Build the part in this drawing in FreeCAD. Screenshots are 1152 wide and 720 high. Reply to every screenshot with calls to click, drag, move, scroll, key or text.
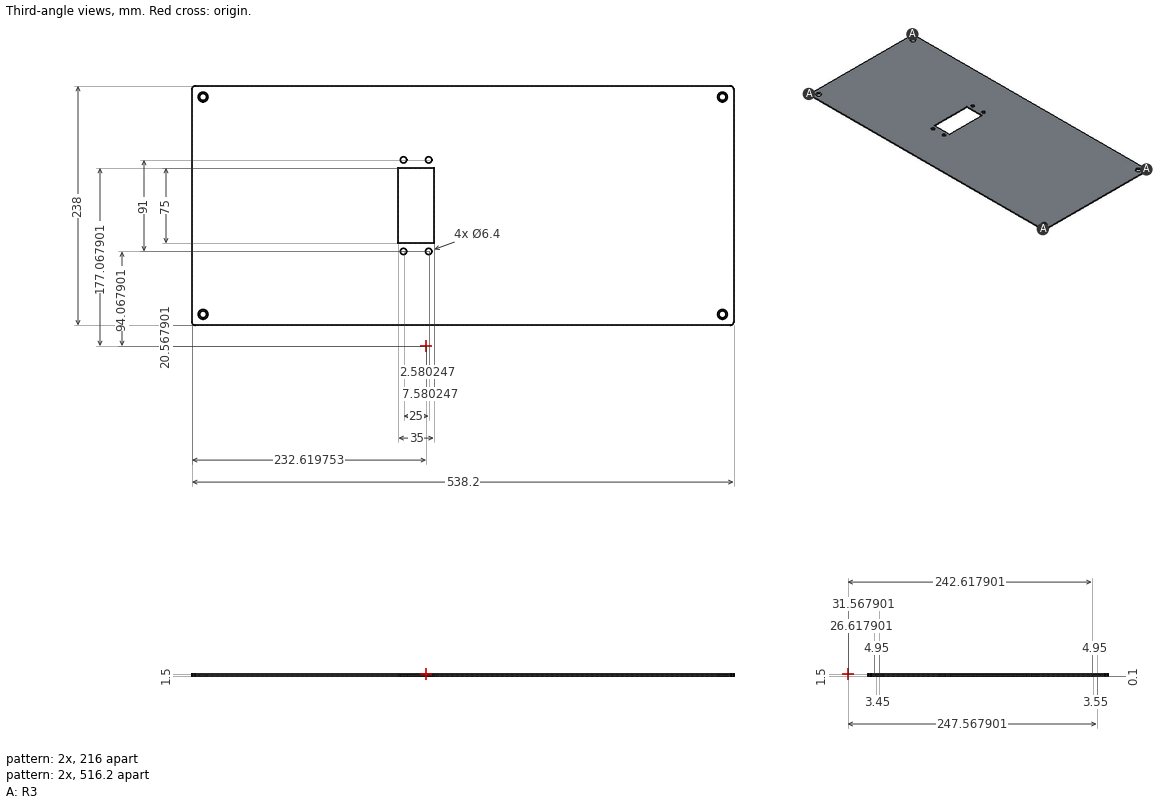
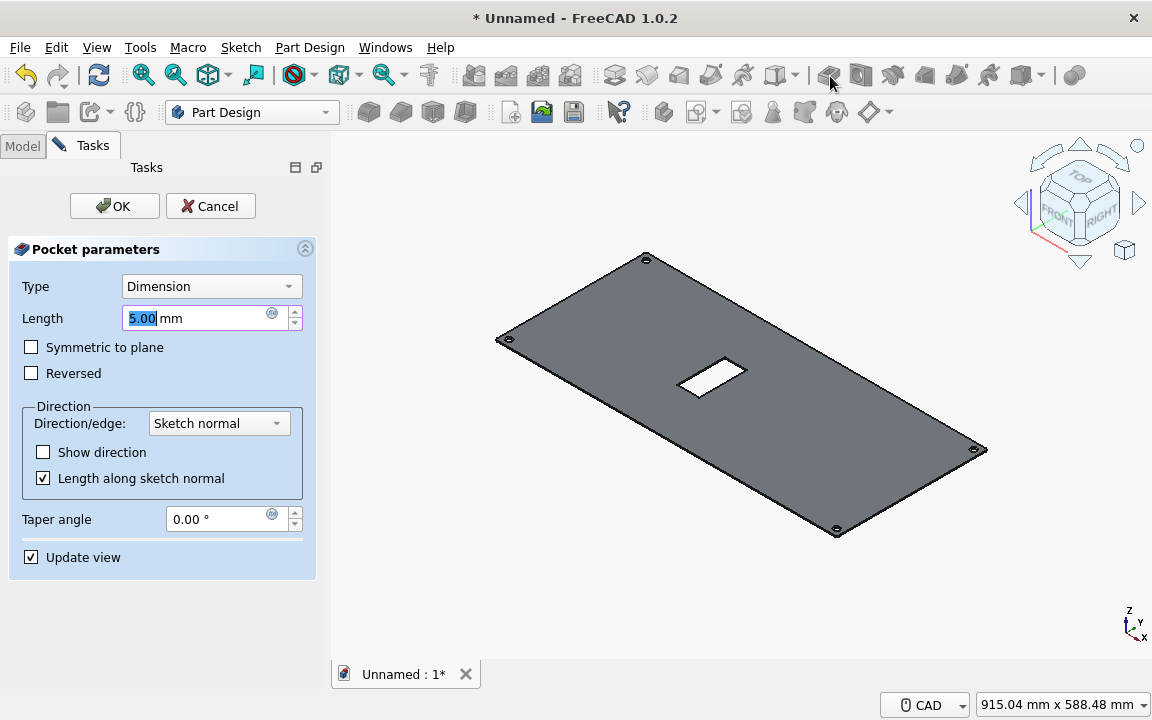
text(1.5)
key(Tab)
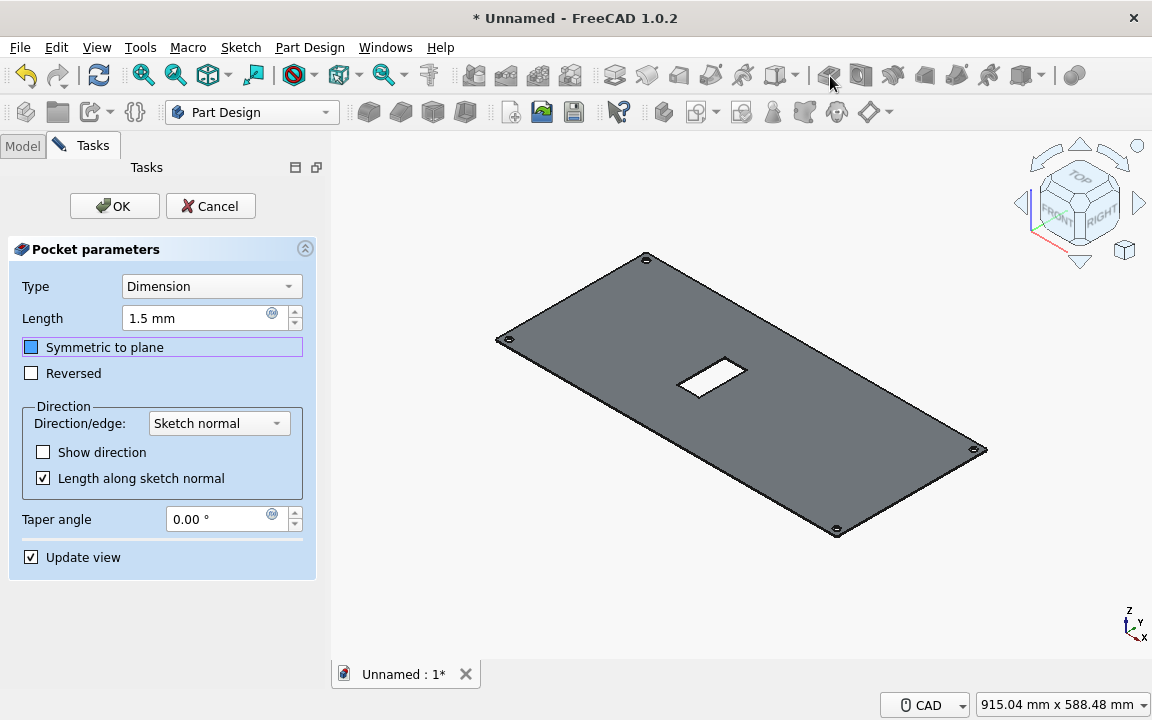
click(115, 206)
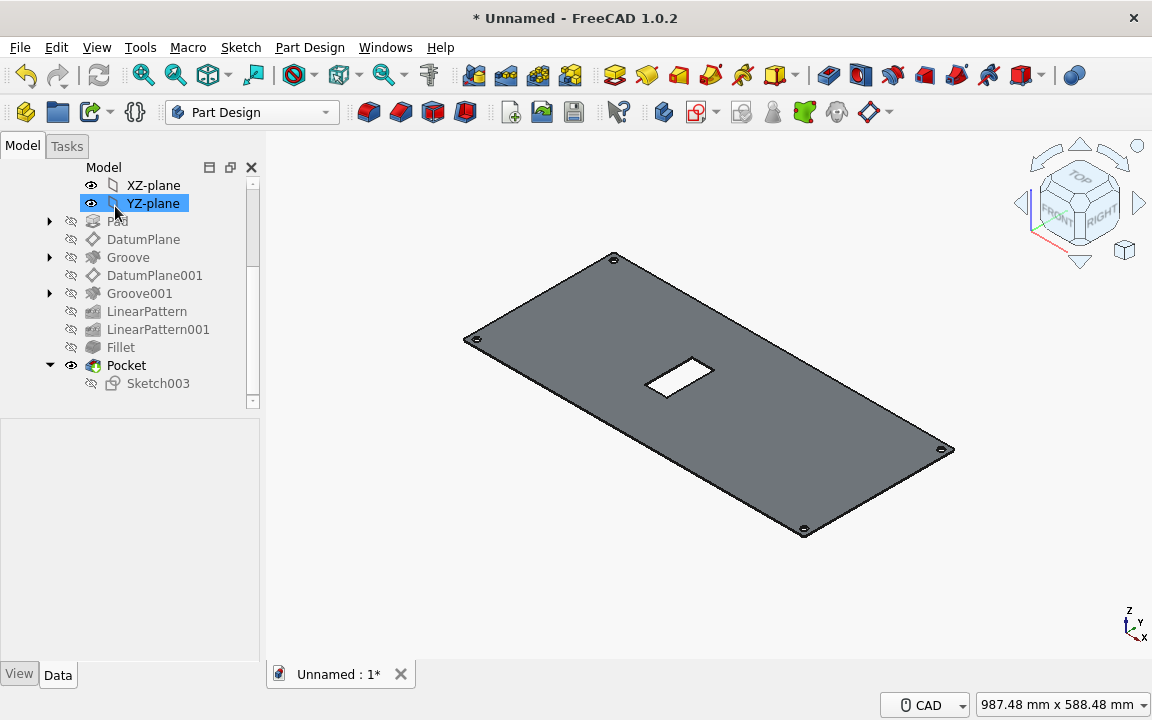
click(807, 450)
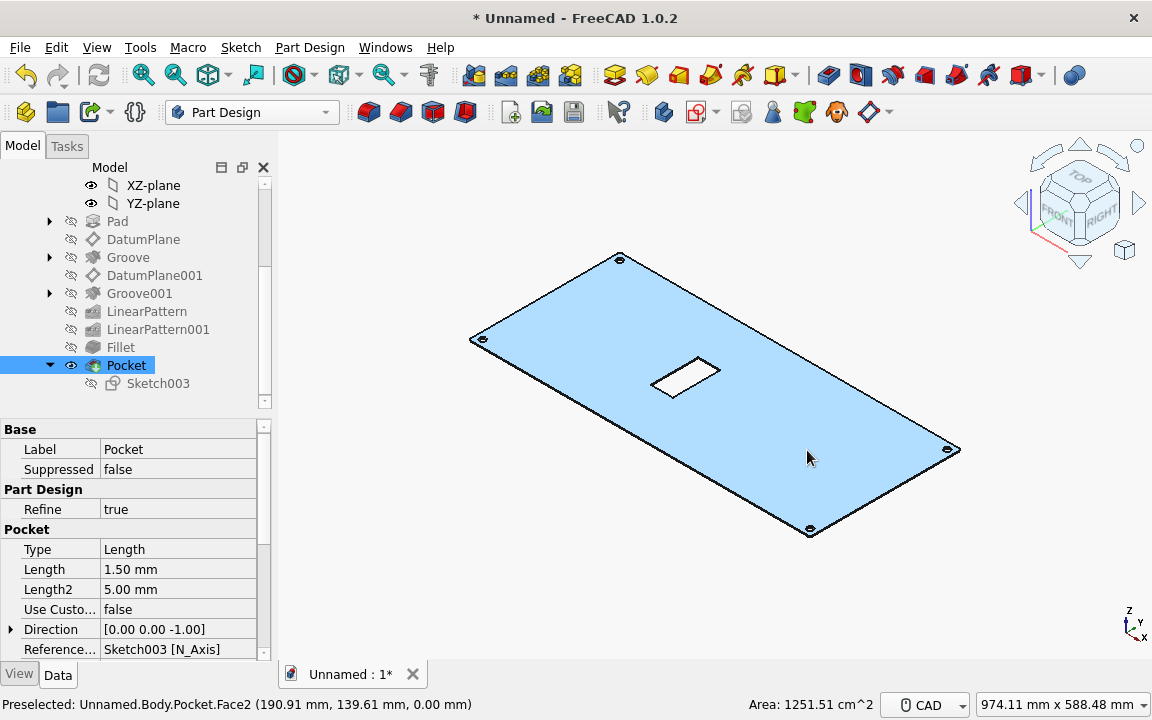
click(696, 112)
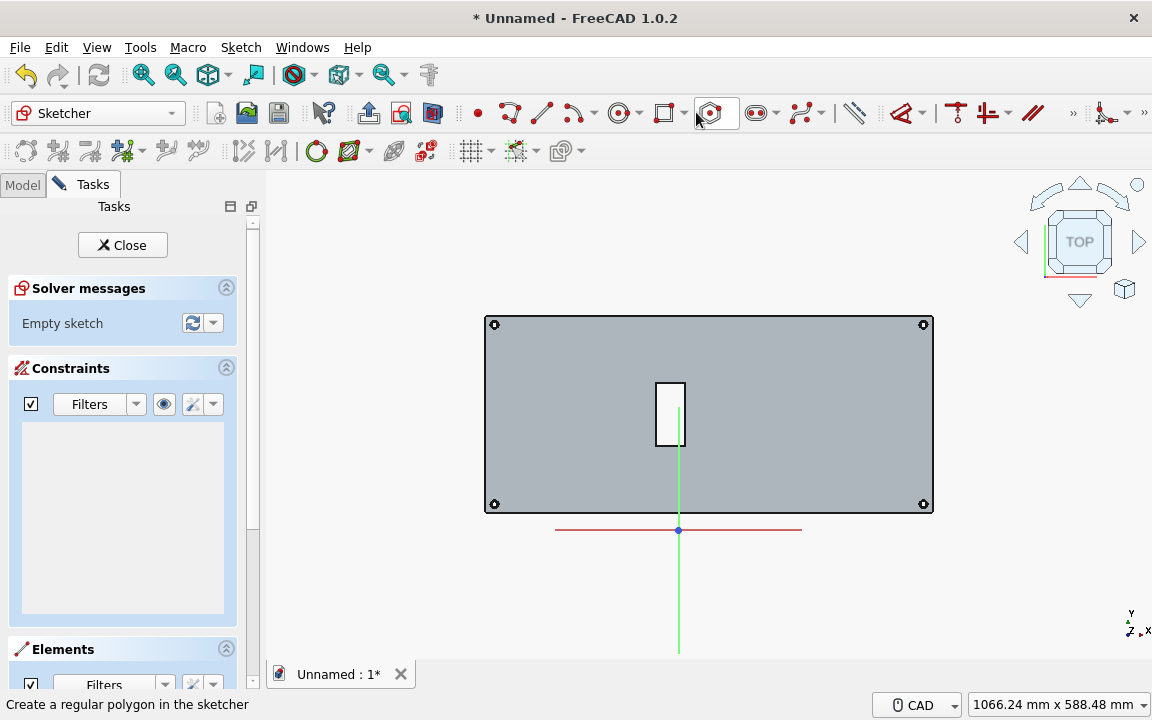
scroll(707, 498, up, 3)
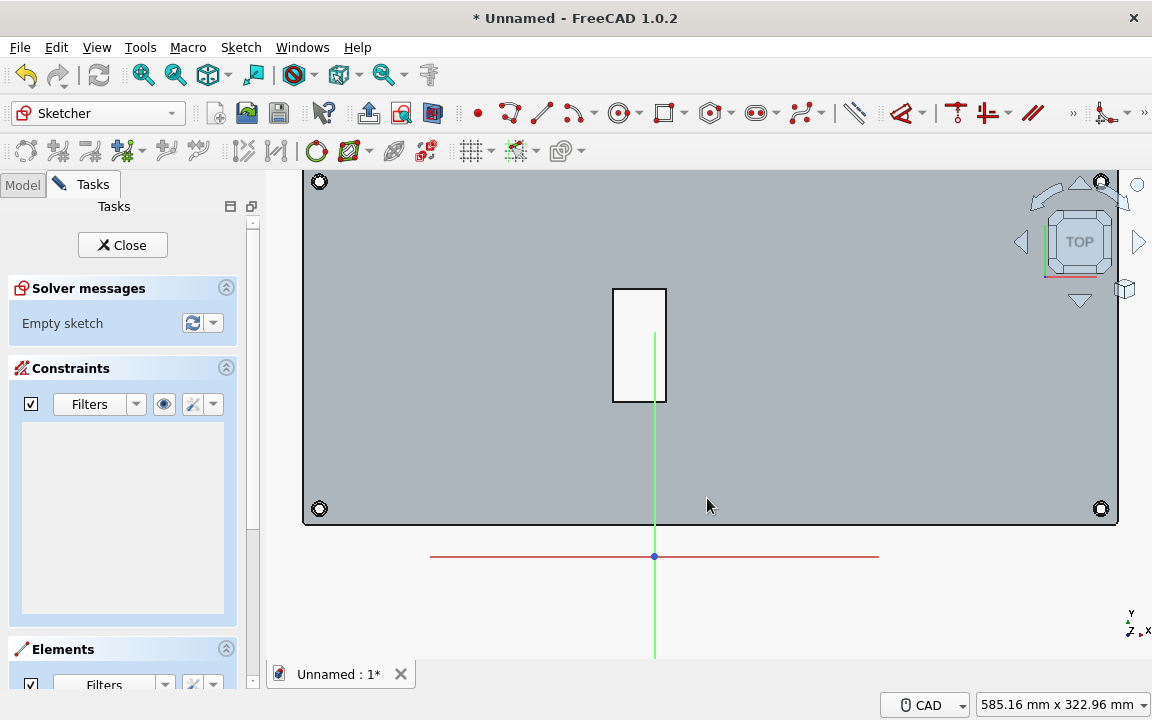
key(g)
key(c)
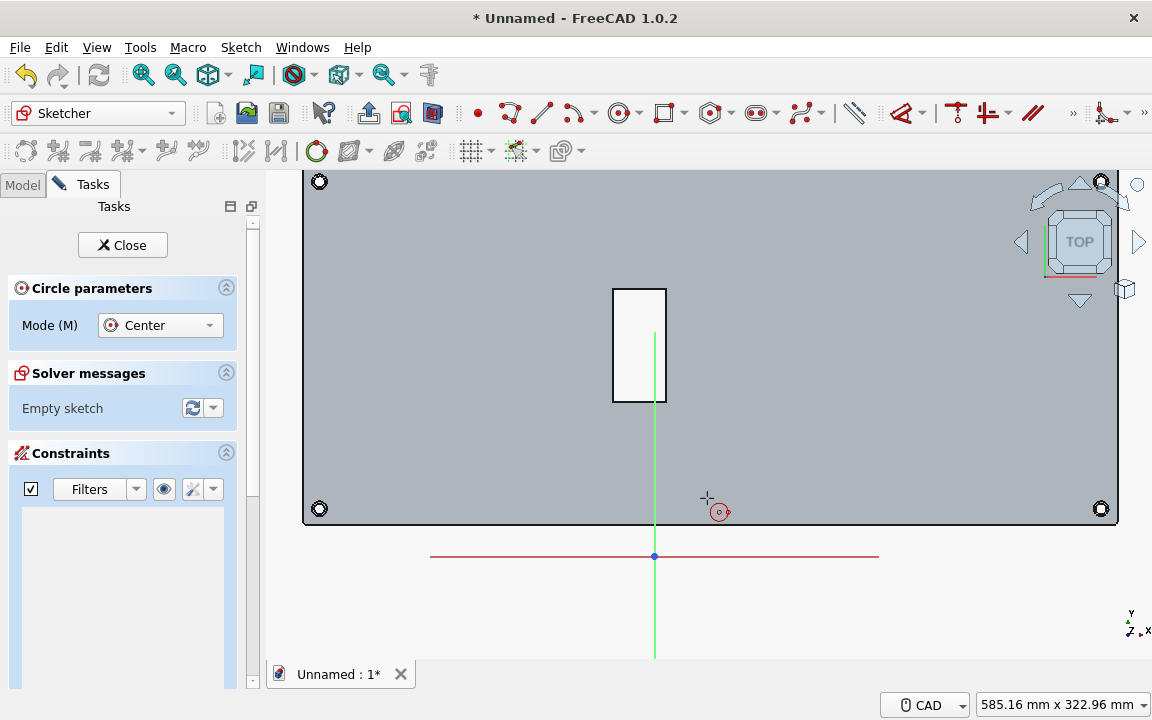
scroll(659, 414, up, 8)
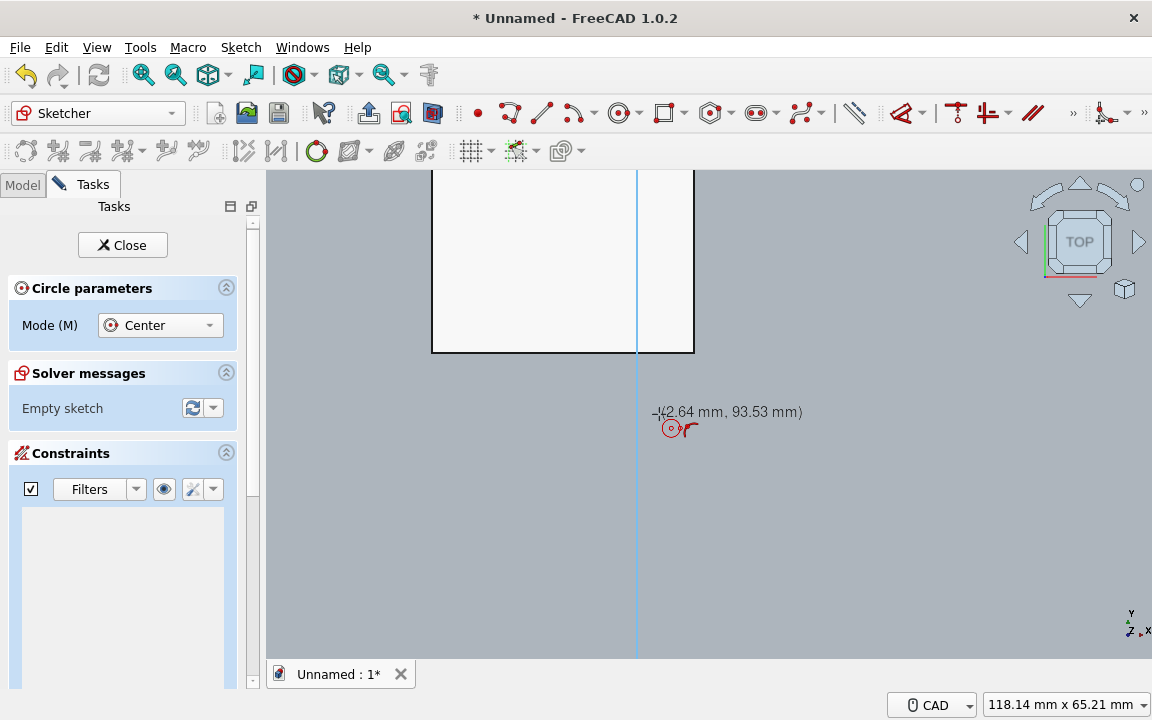
click(657, 413)
click(674, 396)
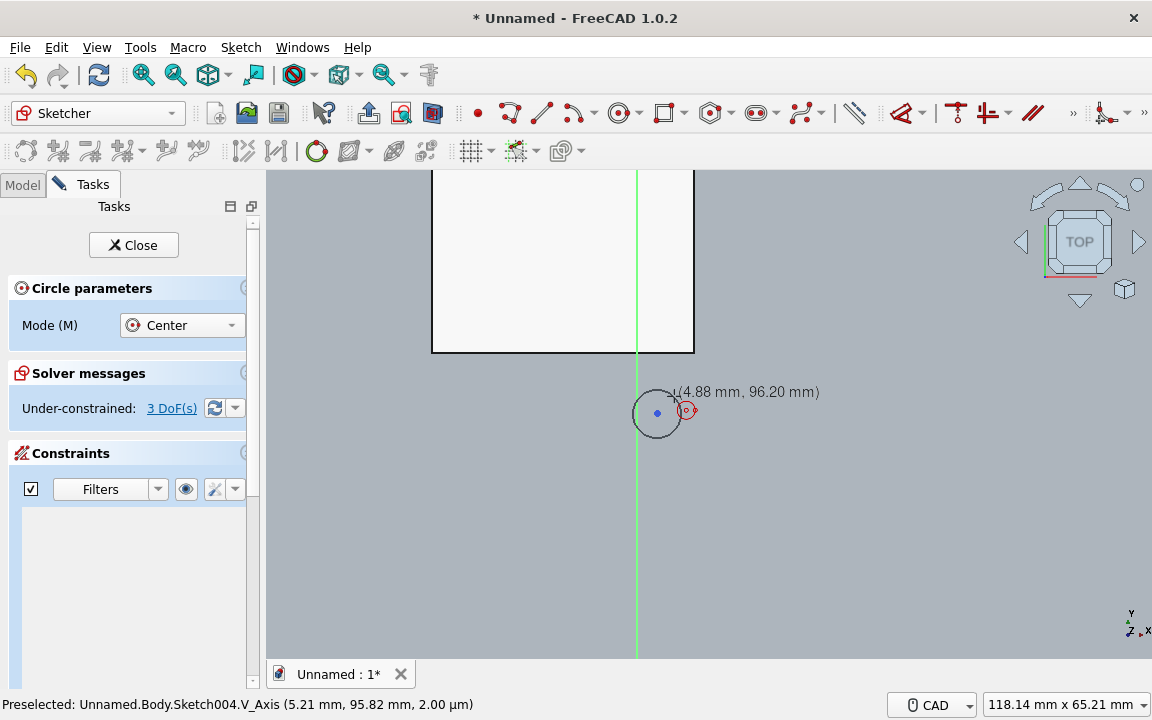
scroll(660, 415, down, 8)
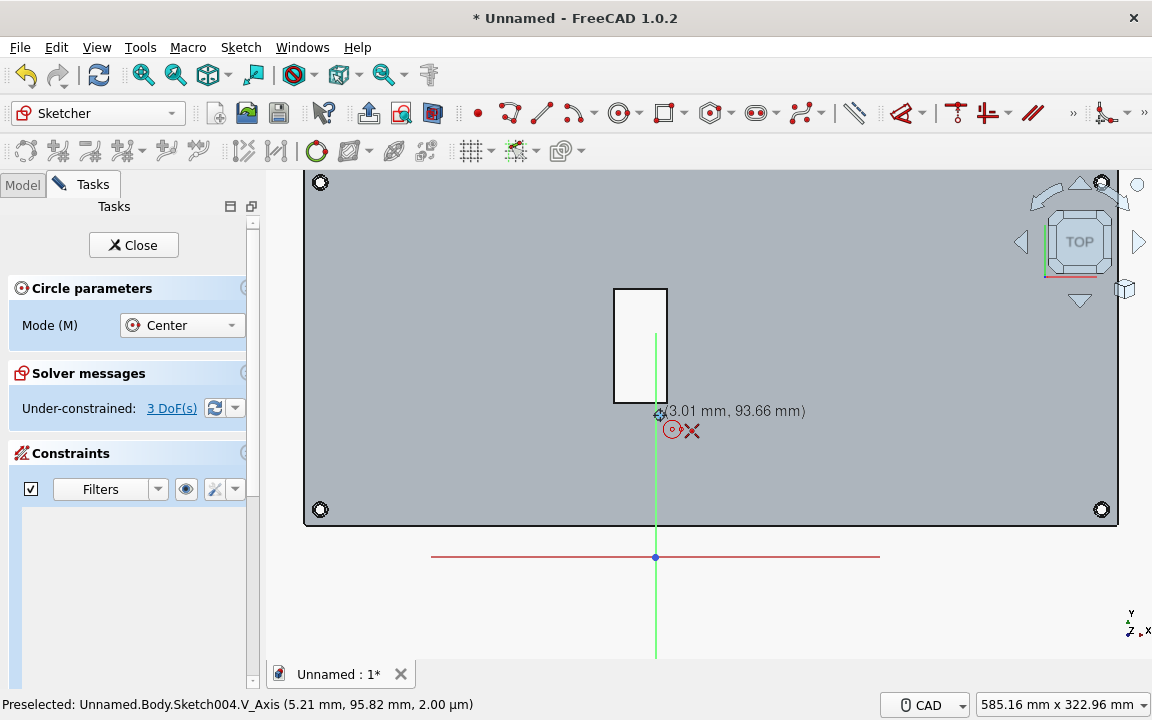
click(622, 415)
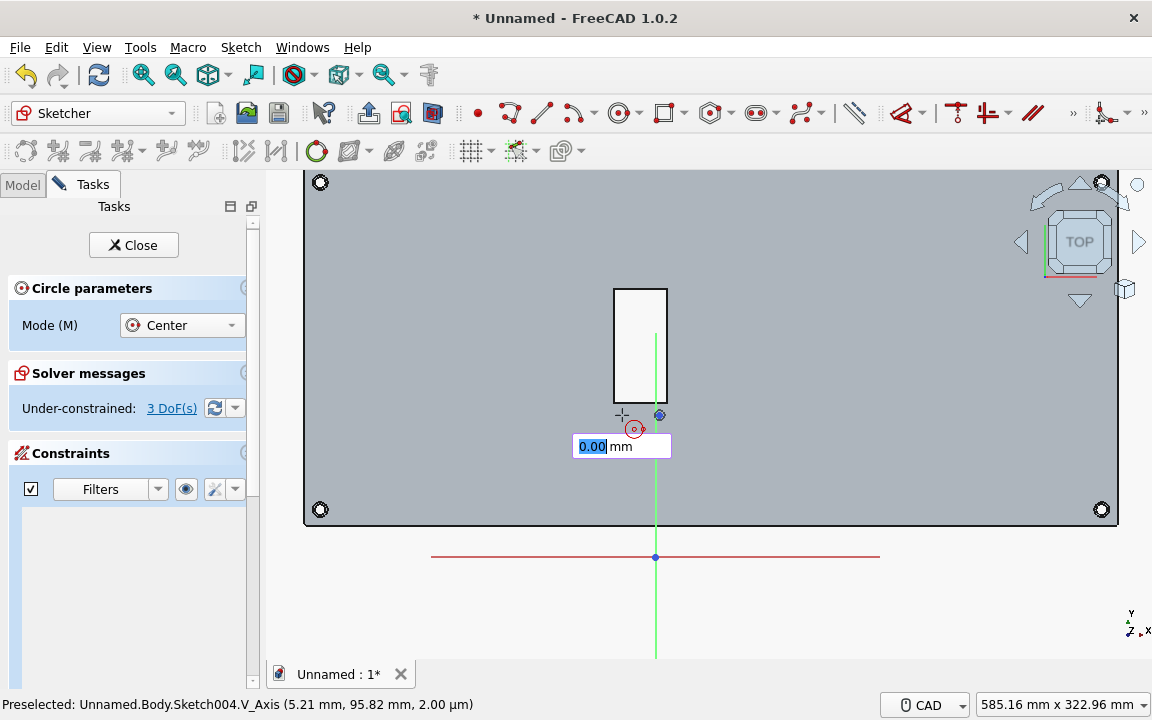
scroll(625, 412, up, 6)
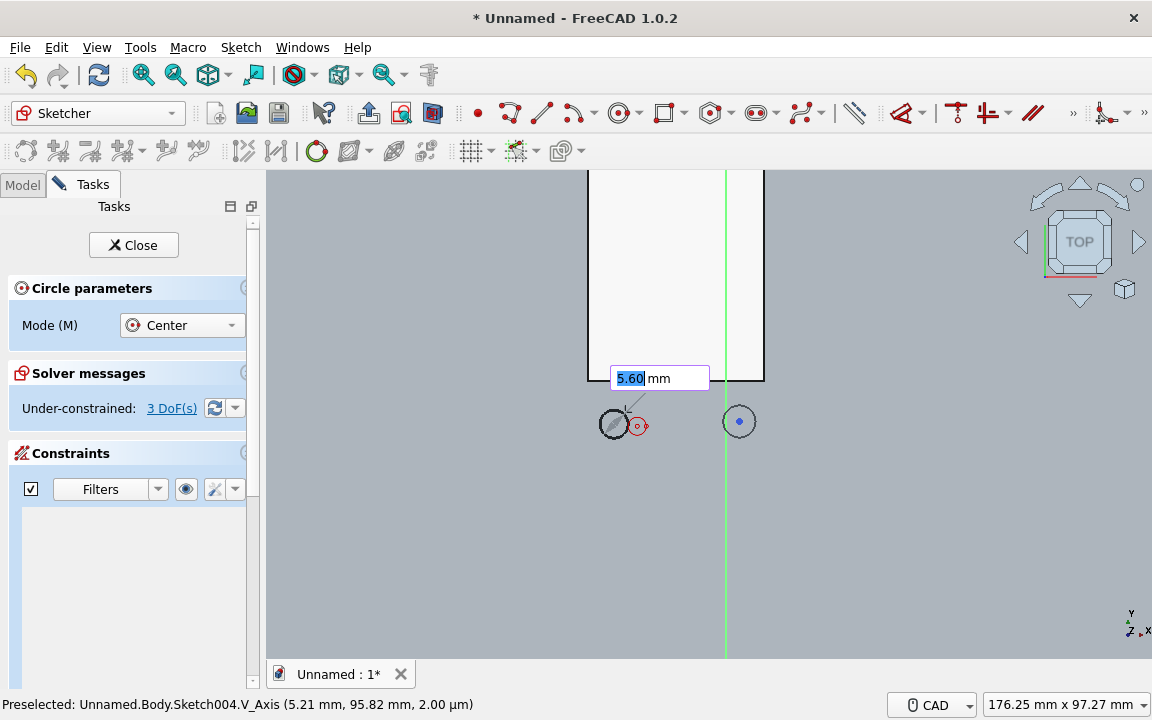
click(625, 409)